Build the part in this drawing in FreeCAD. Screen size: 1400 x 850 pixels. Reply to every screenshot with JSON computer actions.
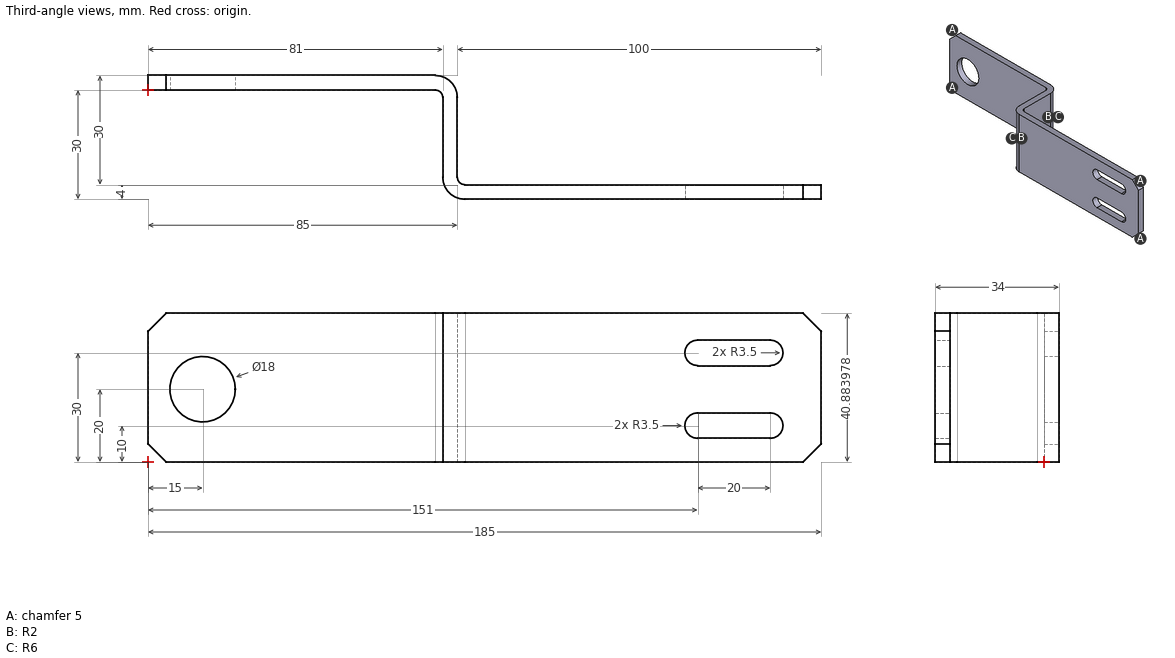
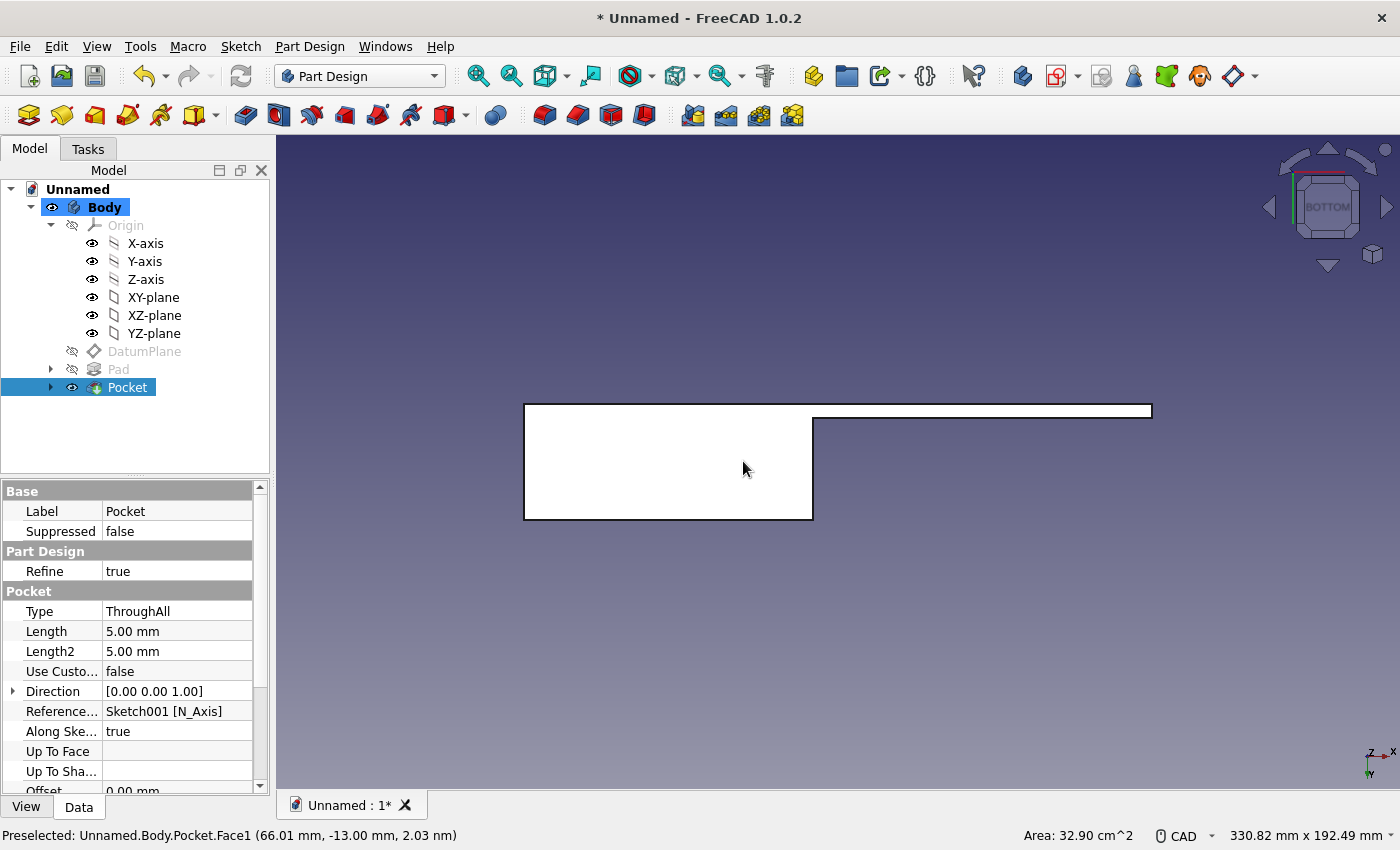
{"action": "left_click", "coordinate": [1056, 76]}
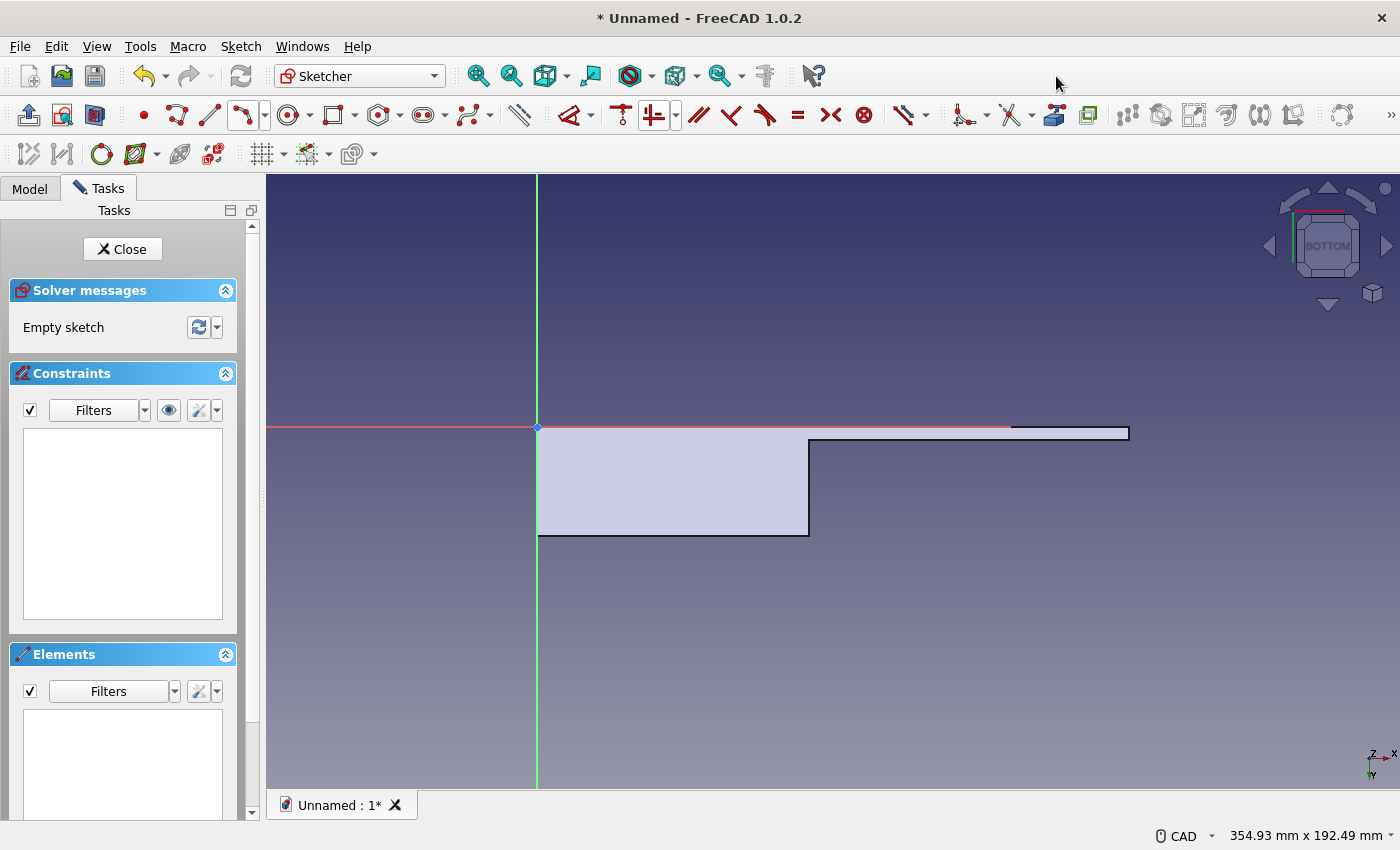
{"action": "scroll", "coordinate": [610, 471], "scroll_direction": "up", "scroll_amount": 5}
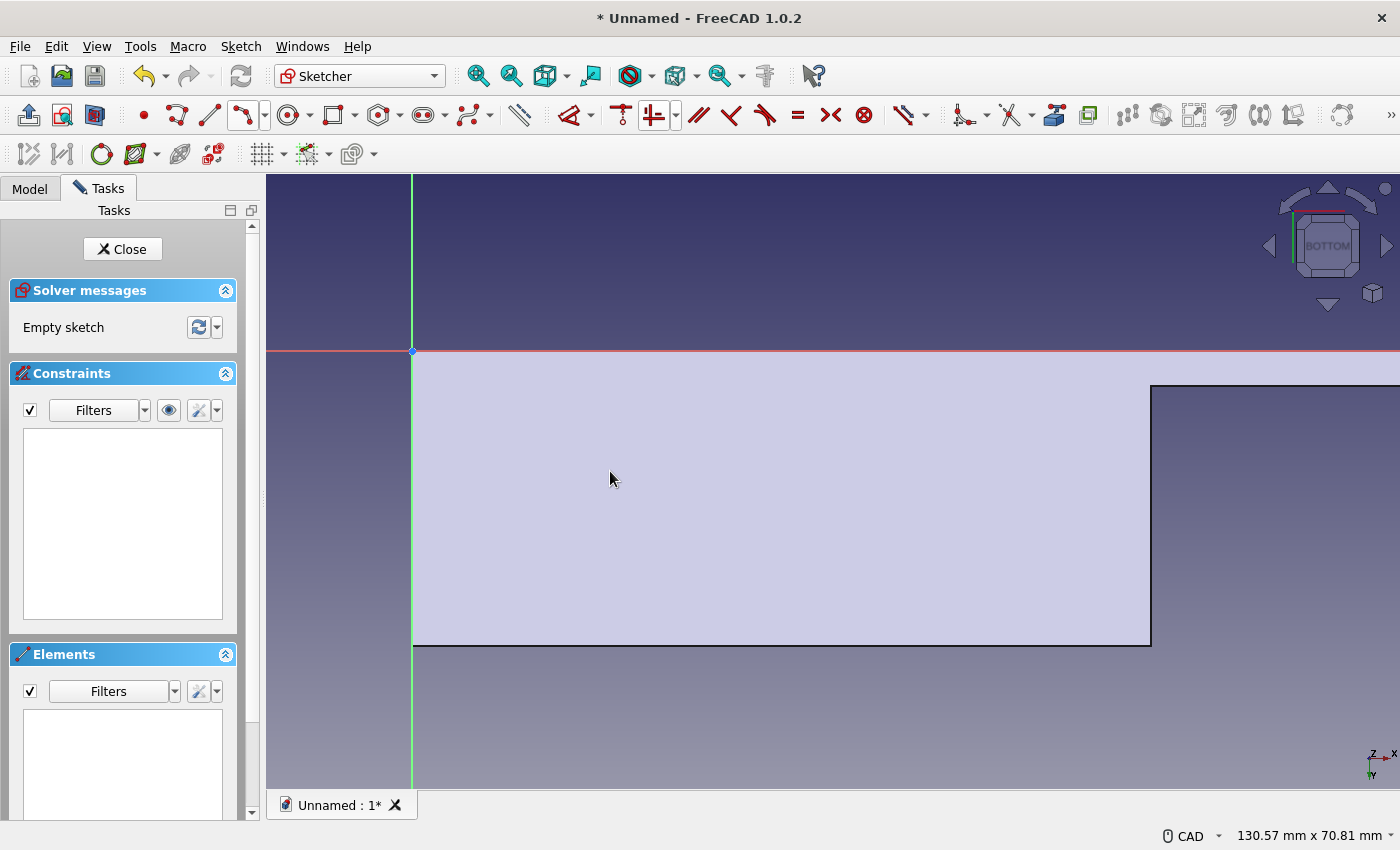
{"action": "left_click", "coordinate": [332, 116]}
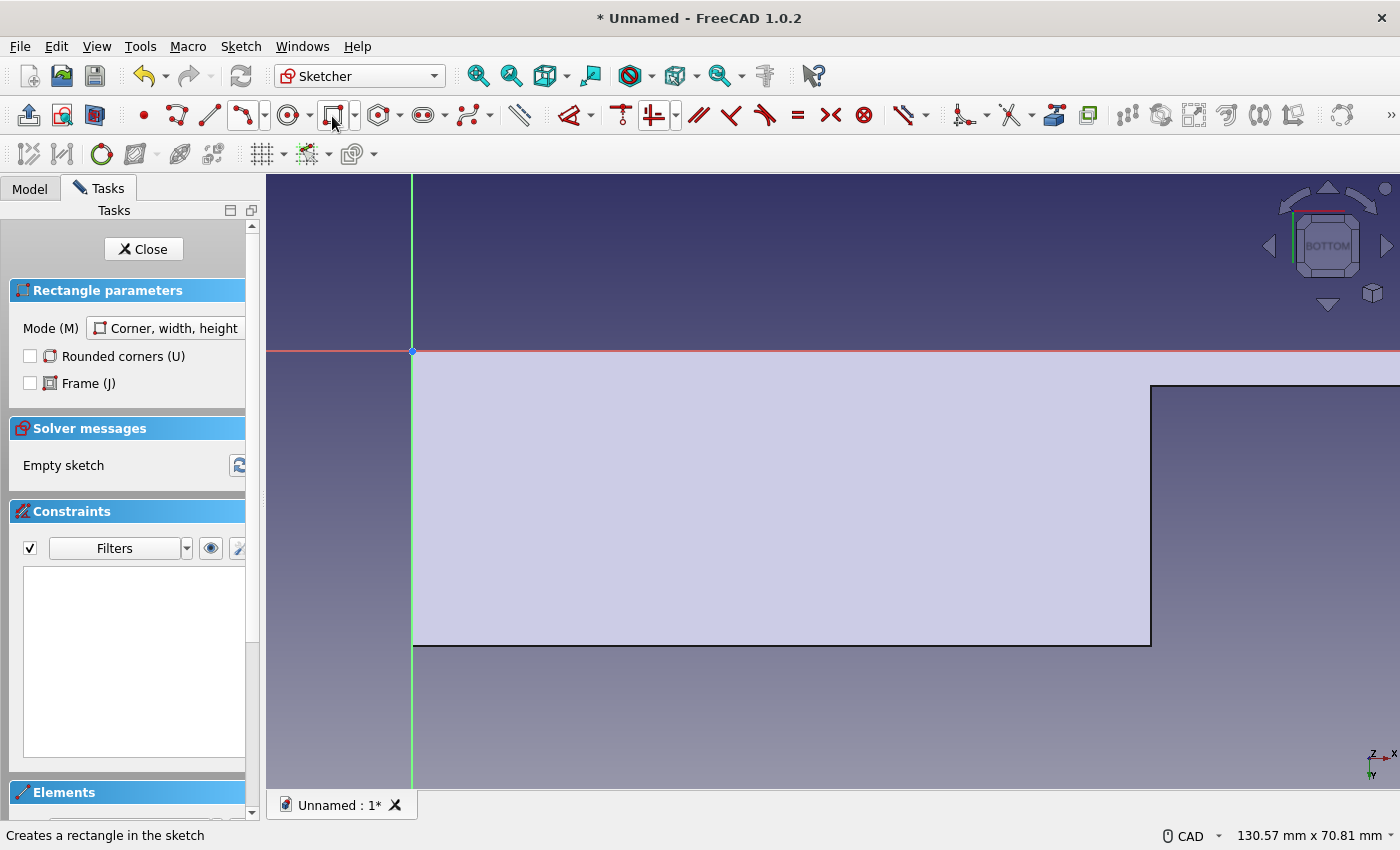
{"action": "left_click", "coordinate": [412, 351]}
{"action": "left_click", "coordinate": [1116, 612]}
{"action": "key", "text": "Escape"}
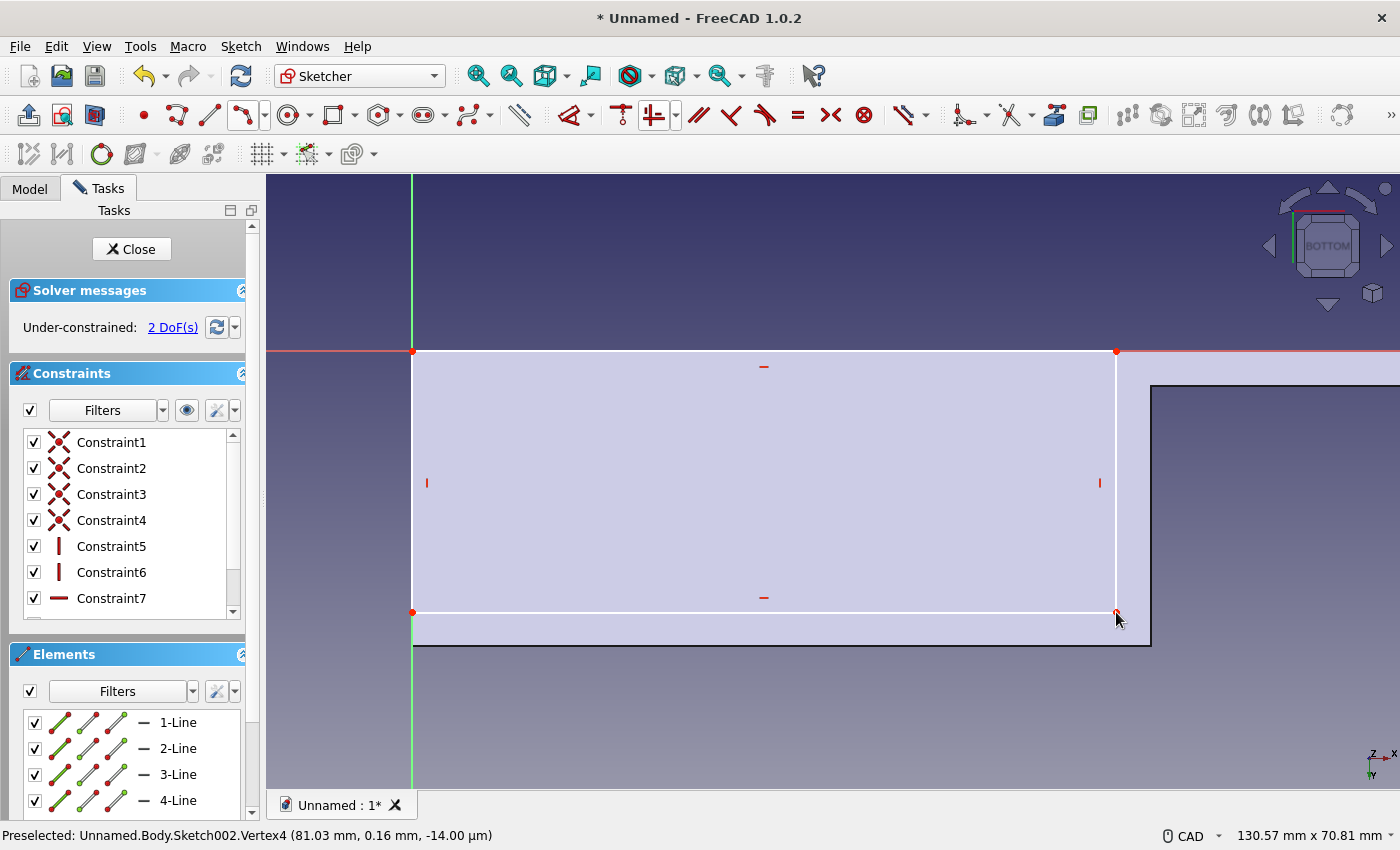
{"action": "left_click", "coordinate": [568, 116]}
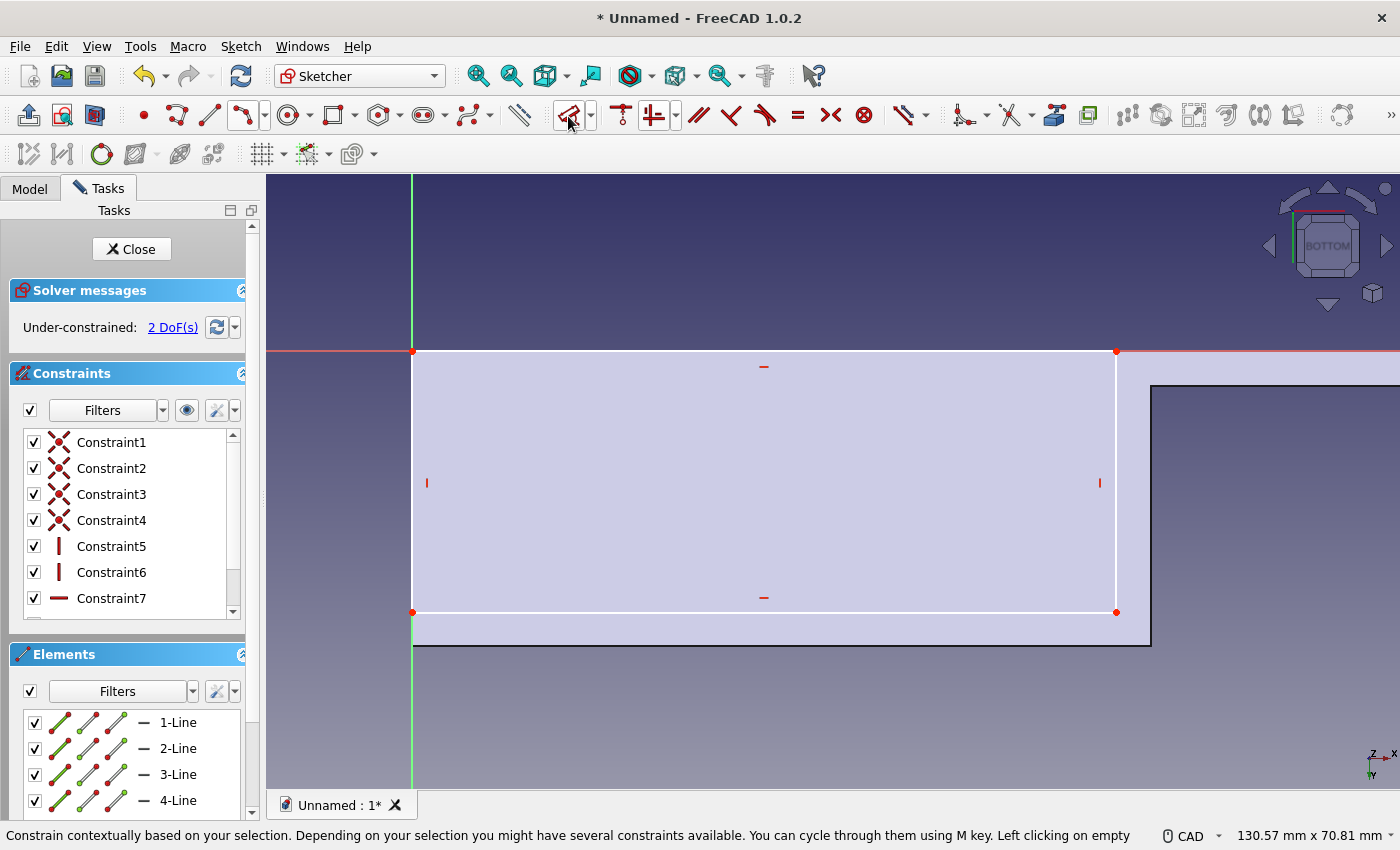
{"action": "left_click", "coordinate": [412, 430]}
{"action": "left_click", "coordinate": [378, 482]}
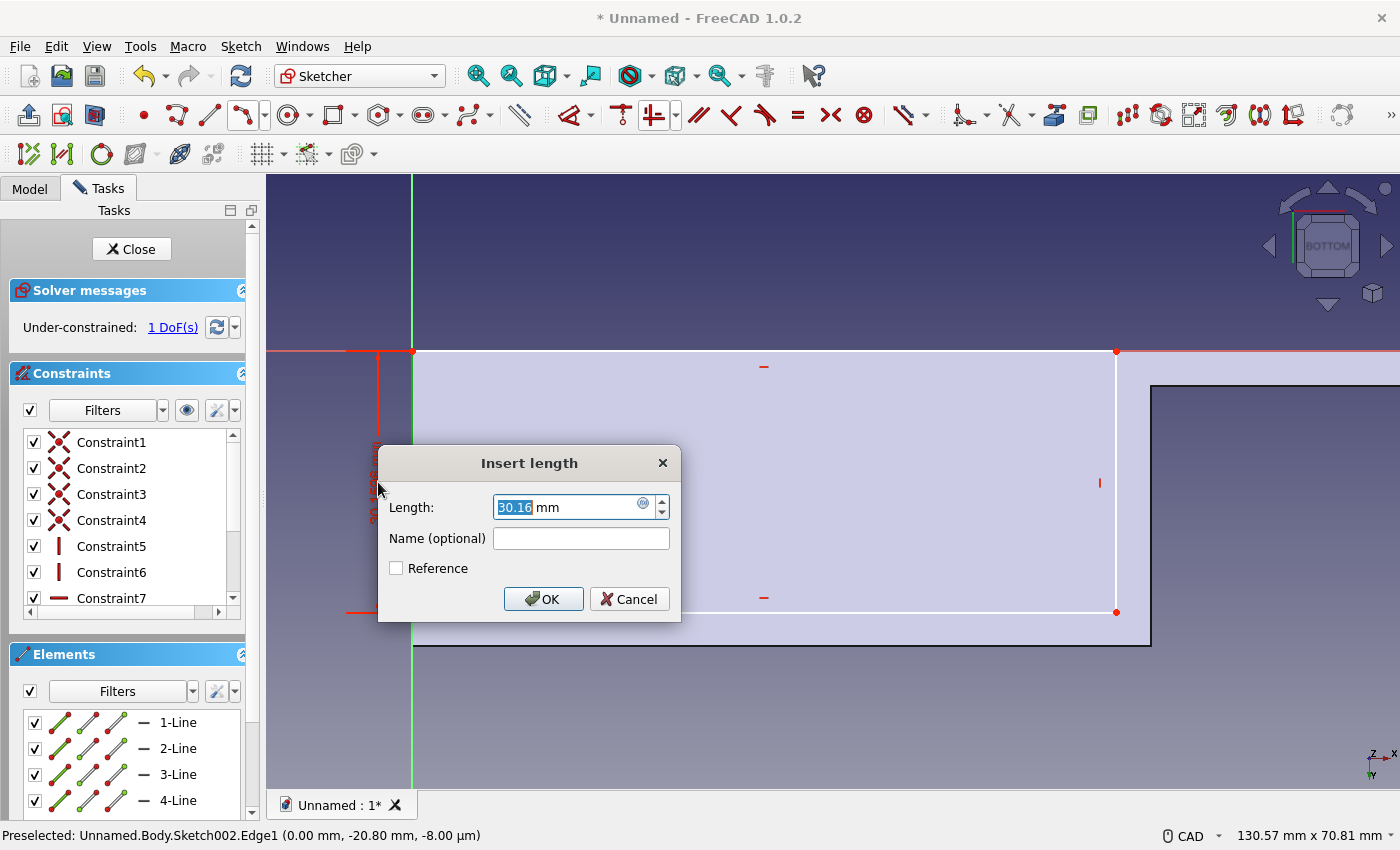
{"action": "type", "text": "30"}
{"action": "key", "text": "Return"}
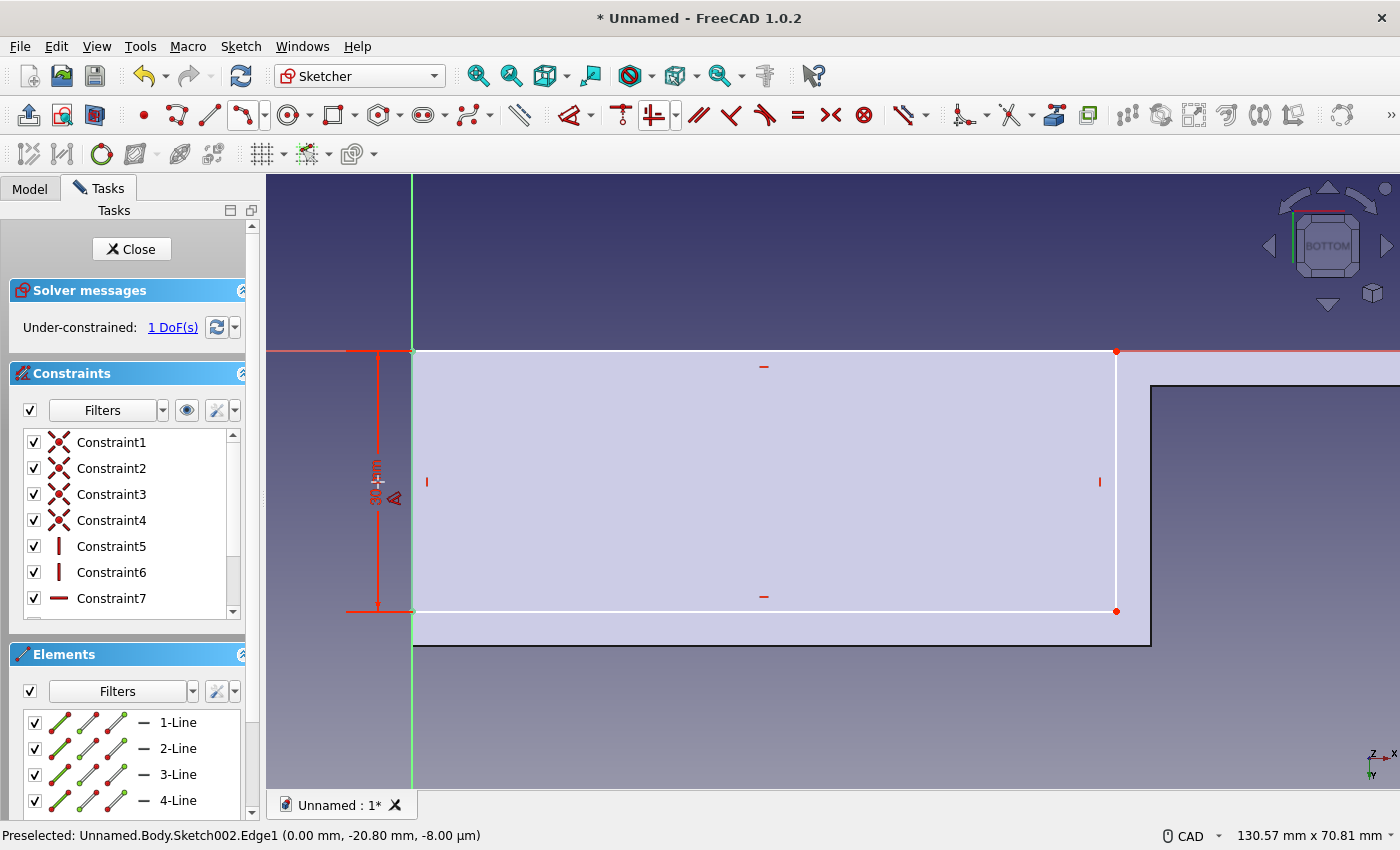
{"action": "left_click", "coordinate": [623, 612]}
{"action": "left_click", "coordinate": [764, 646]}